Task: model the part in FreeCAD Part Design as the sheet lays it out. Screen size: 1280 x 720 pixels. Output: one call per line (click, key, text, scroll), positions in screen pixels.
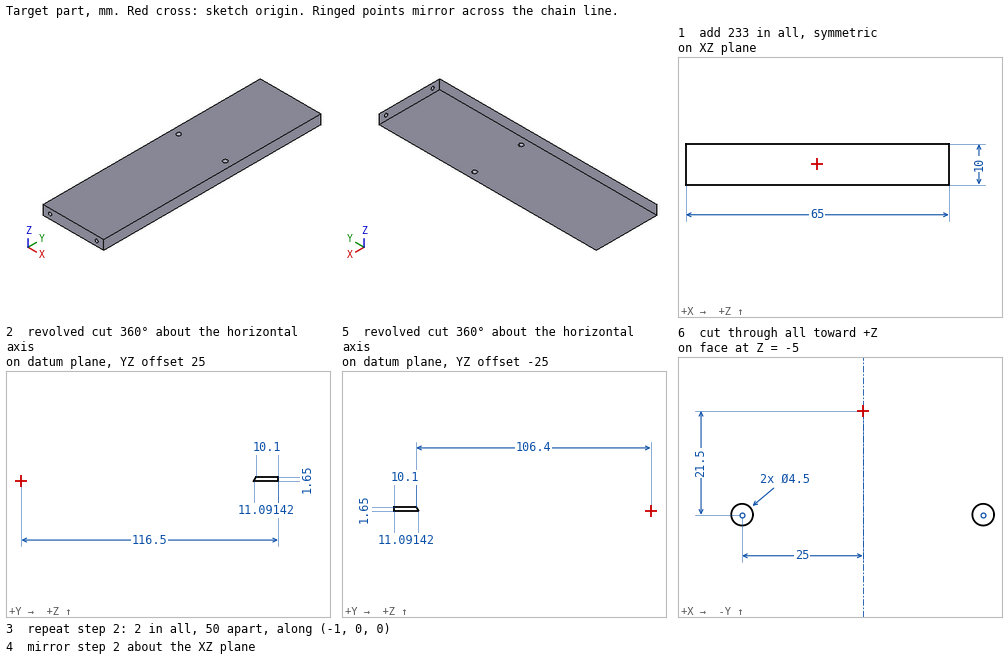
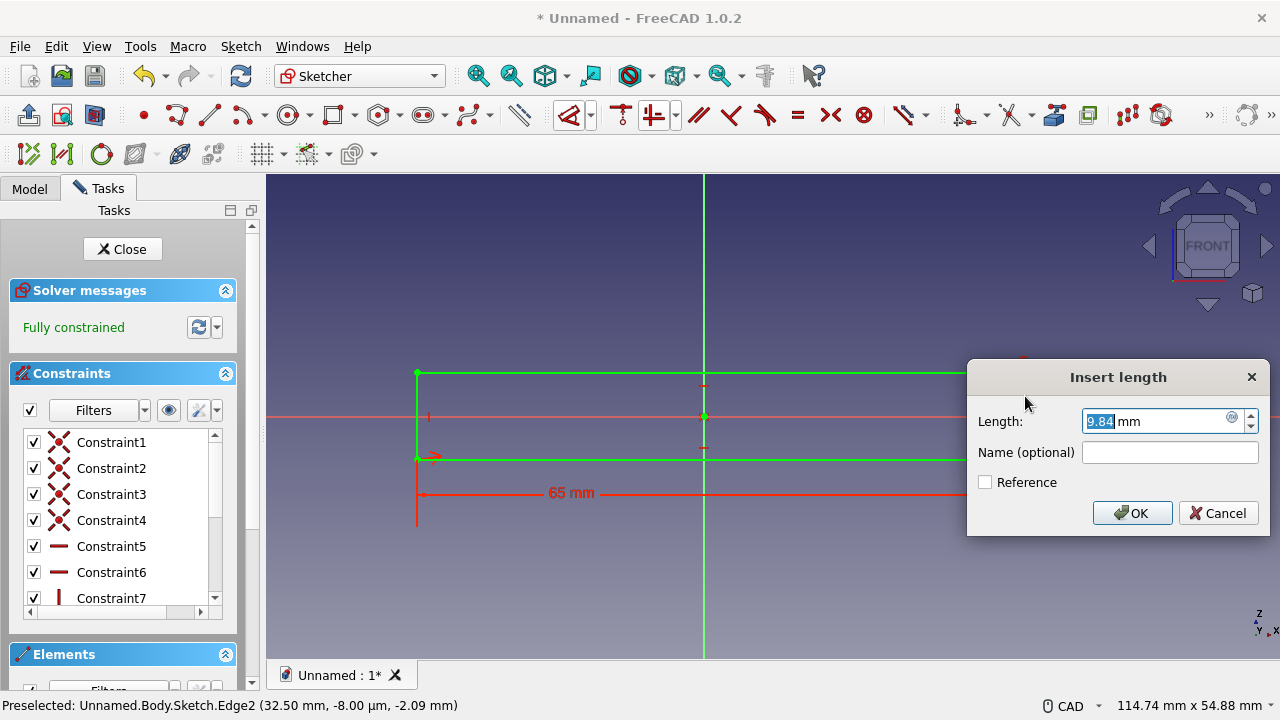
text(10)
key(Return)
key(Escape)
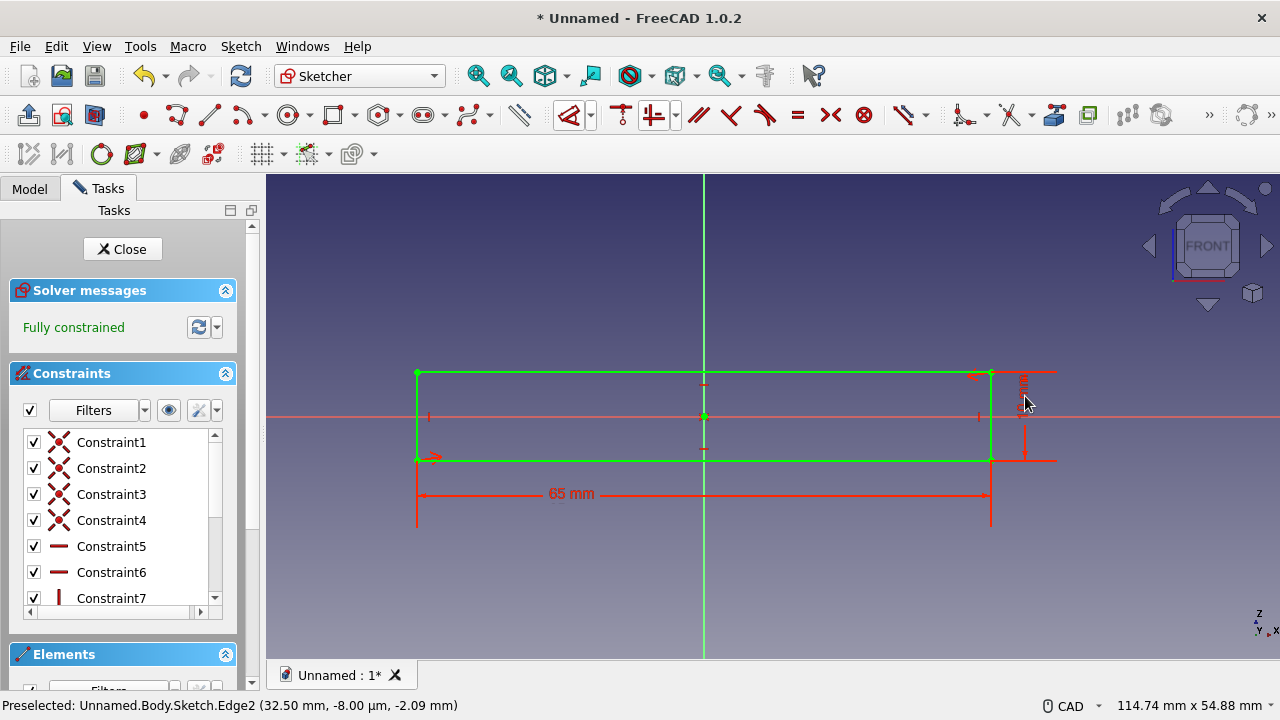
click(123, 249)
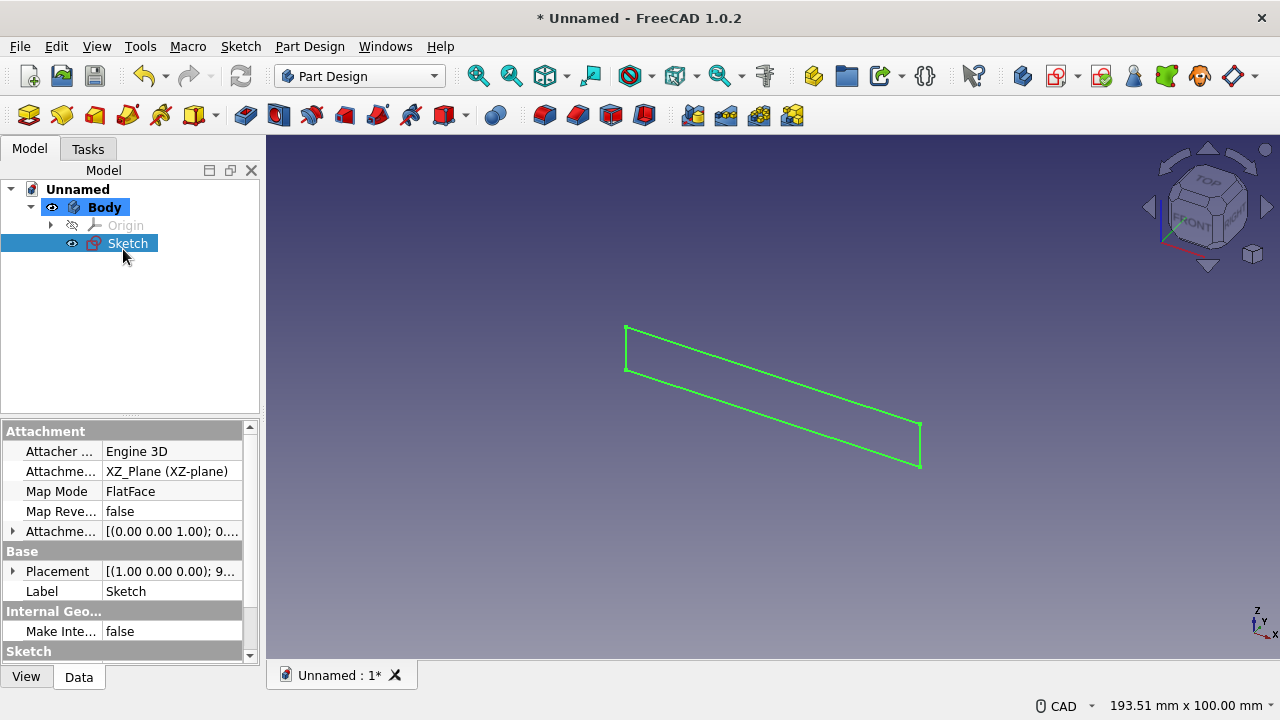
click(29, 116)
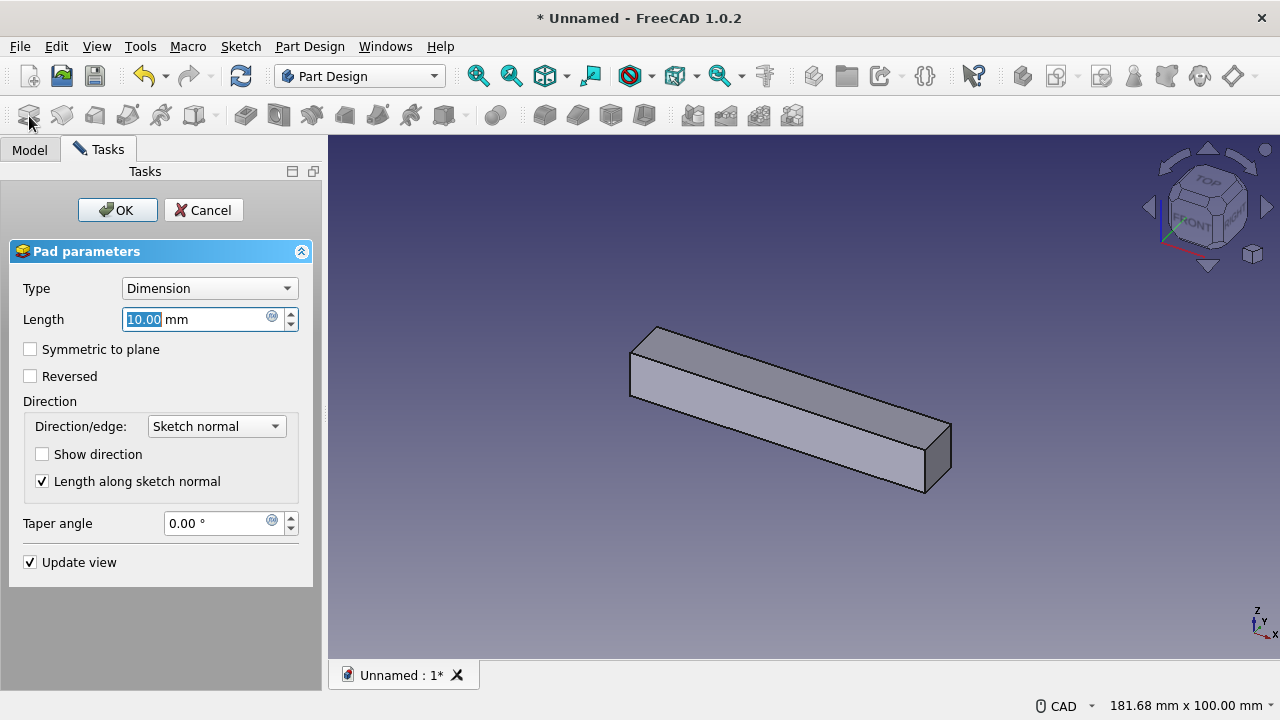
text(233)
key(Tab)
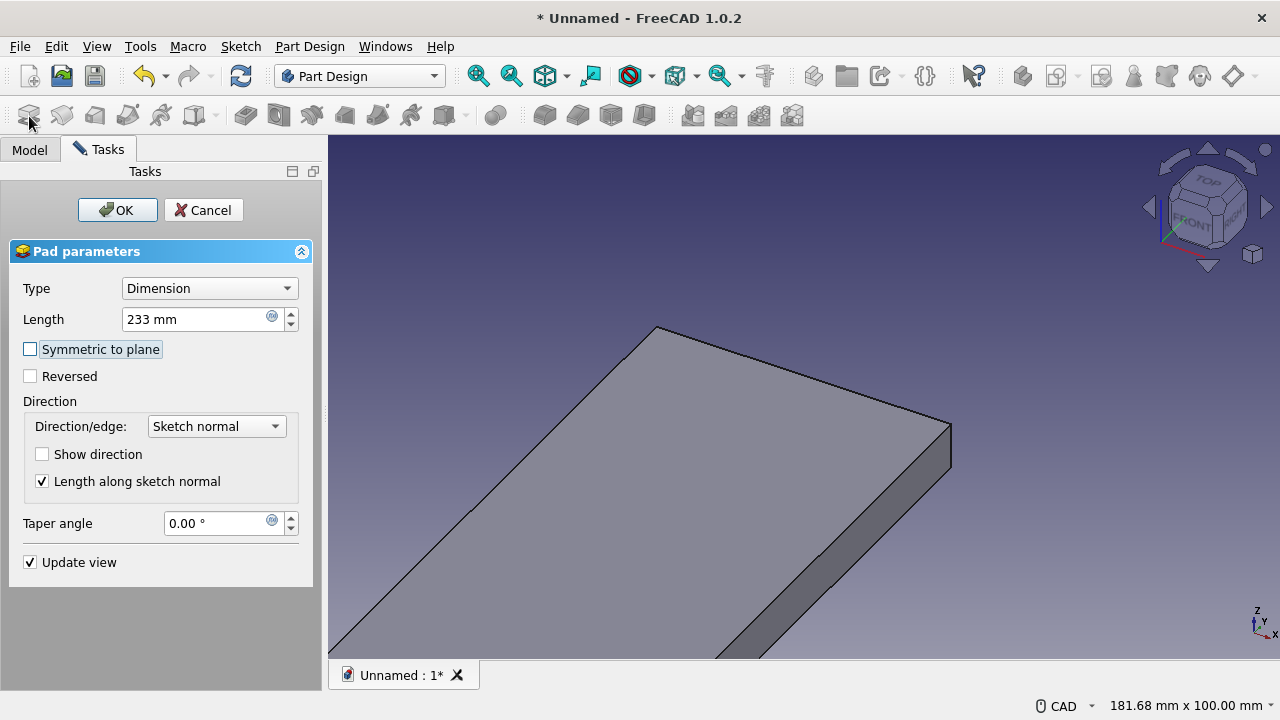
click(31, 349)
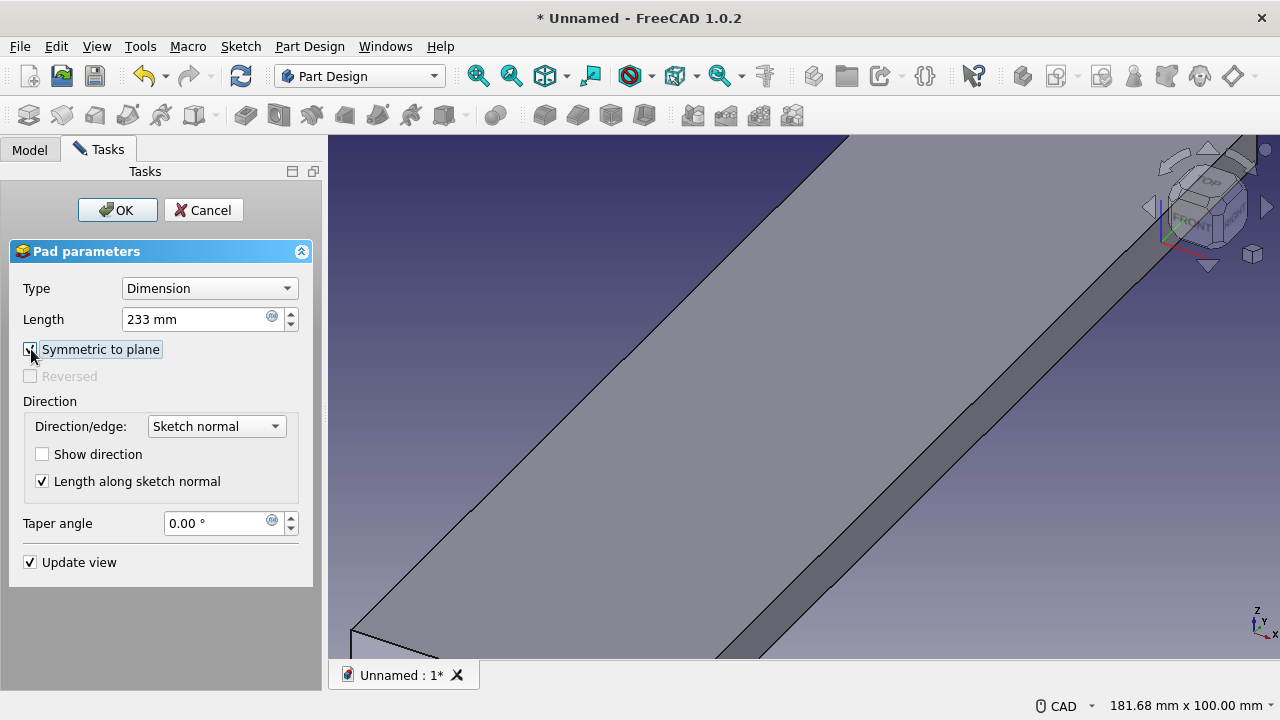
click(118, 210)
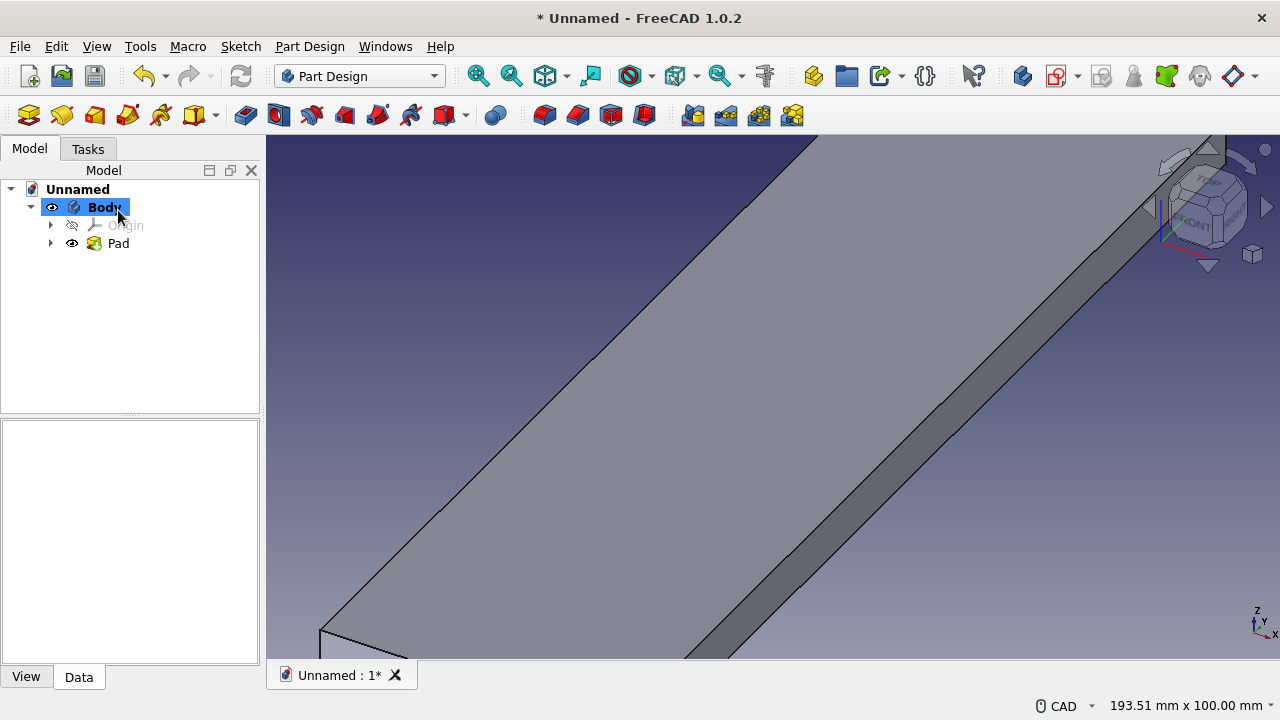
key(v)
key(f)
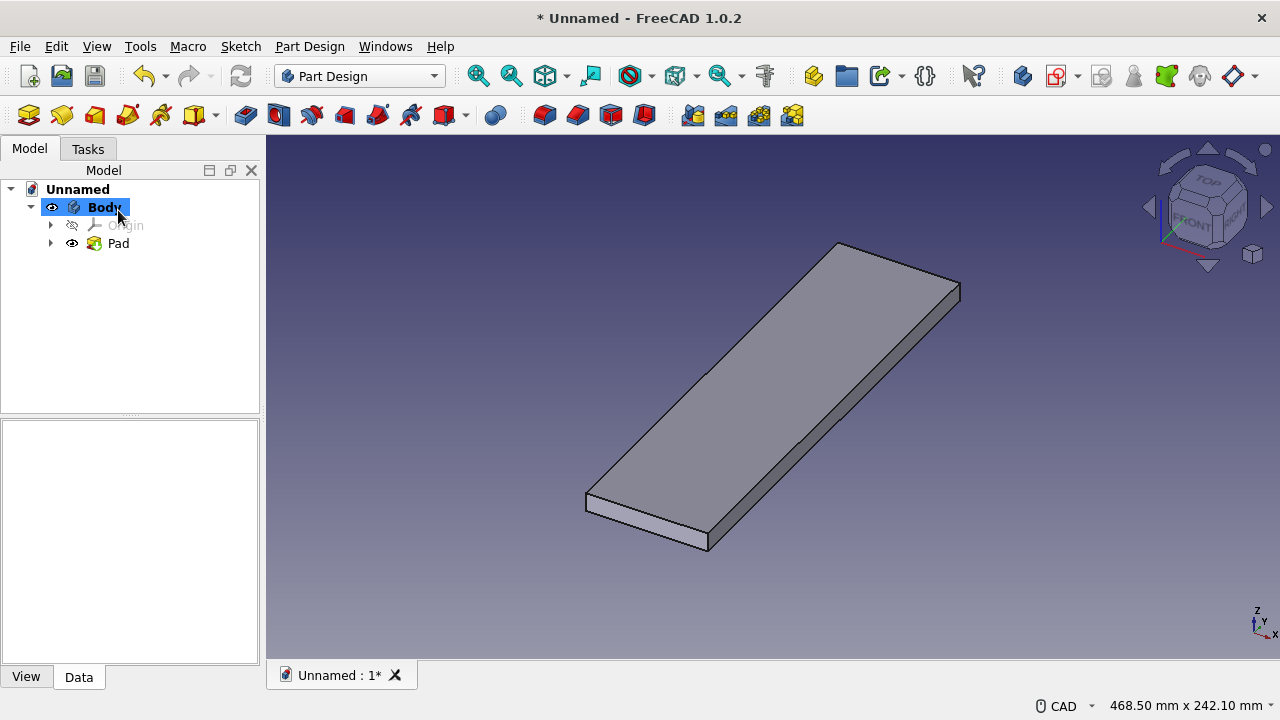
click(51, 225)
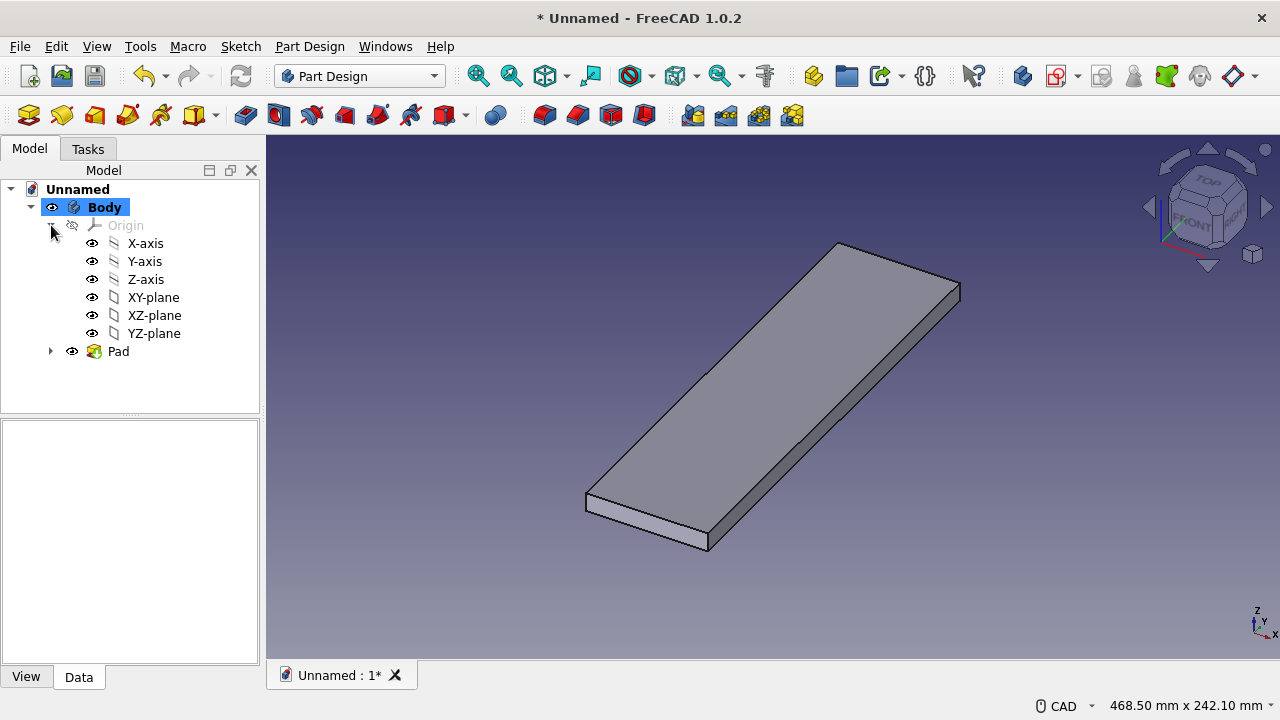
click(137, 333)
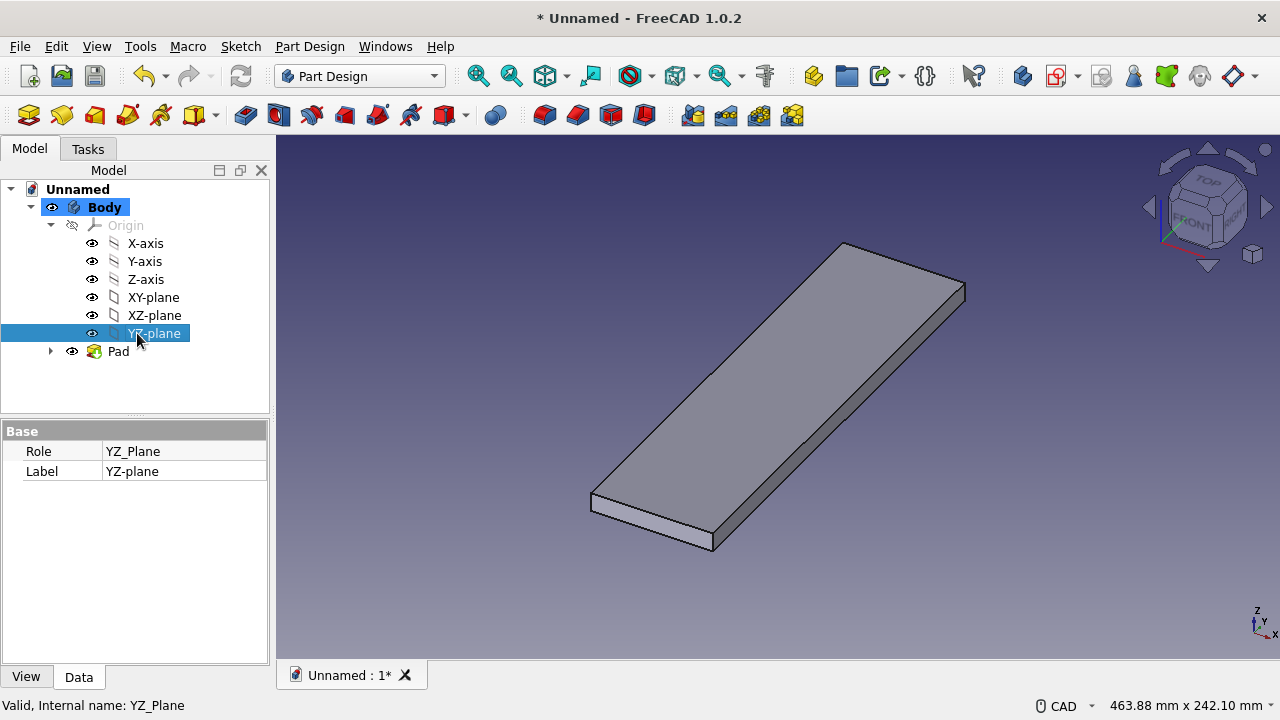
click(1232, 76)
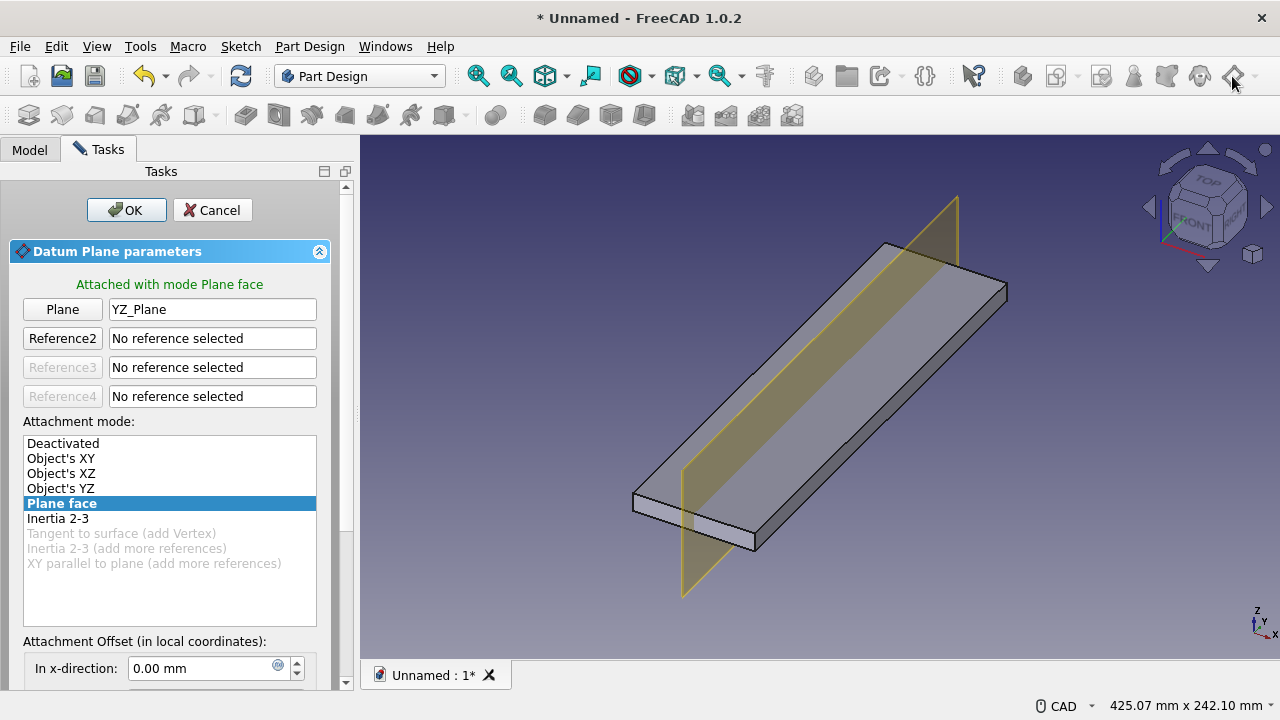
scroll(346, 436, down, 2)